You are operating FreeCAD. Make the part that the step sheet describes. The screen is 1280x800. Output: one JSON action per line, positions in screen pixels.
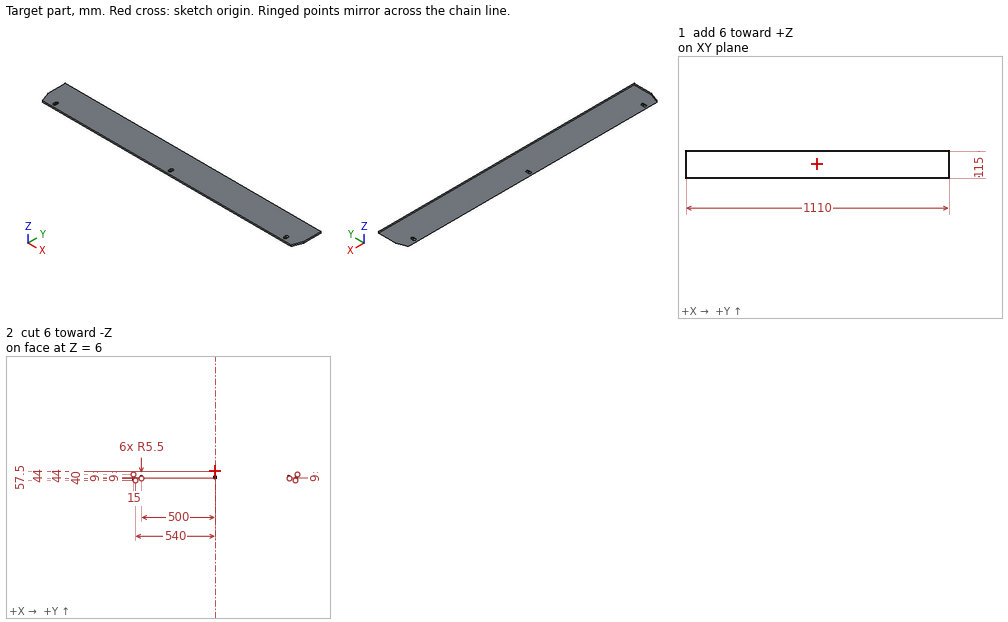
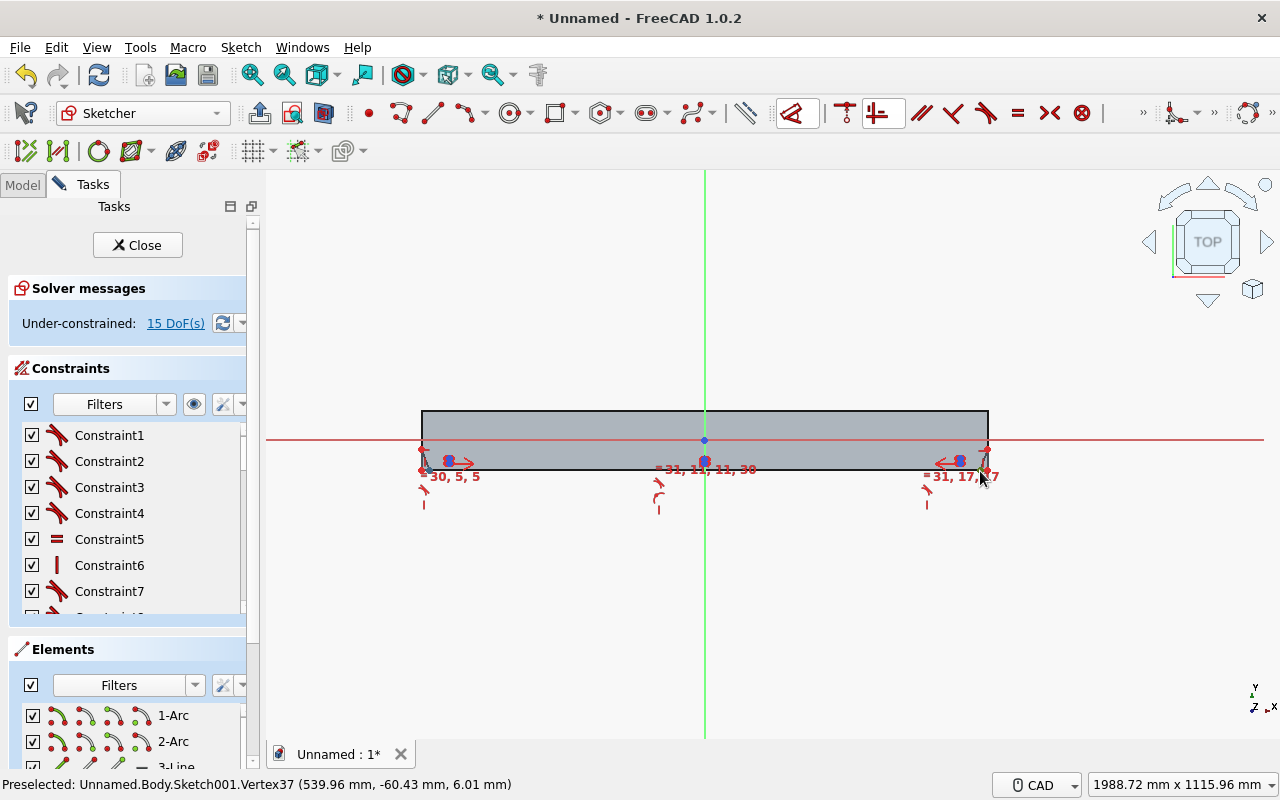
{"action": "left_click", "coordinate": [705, 674]}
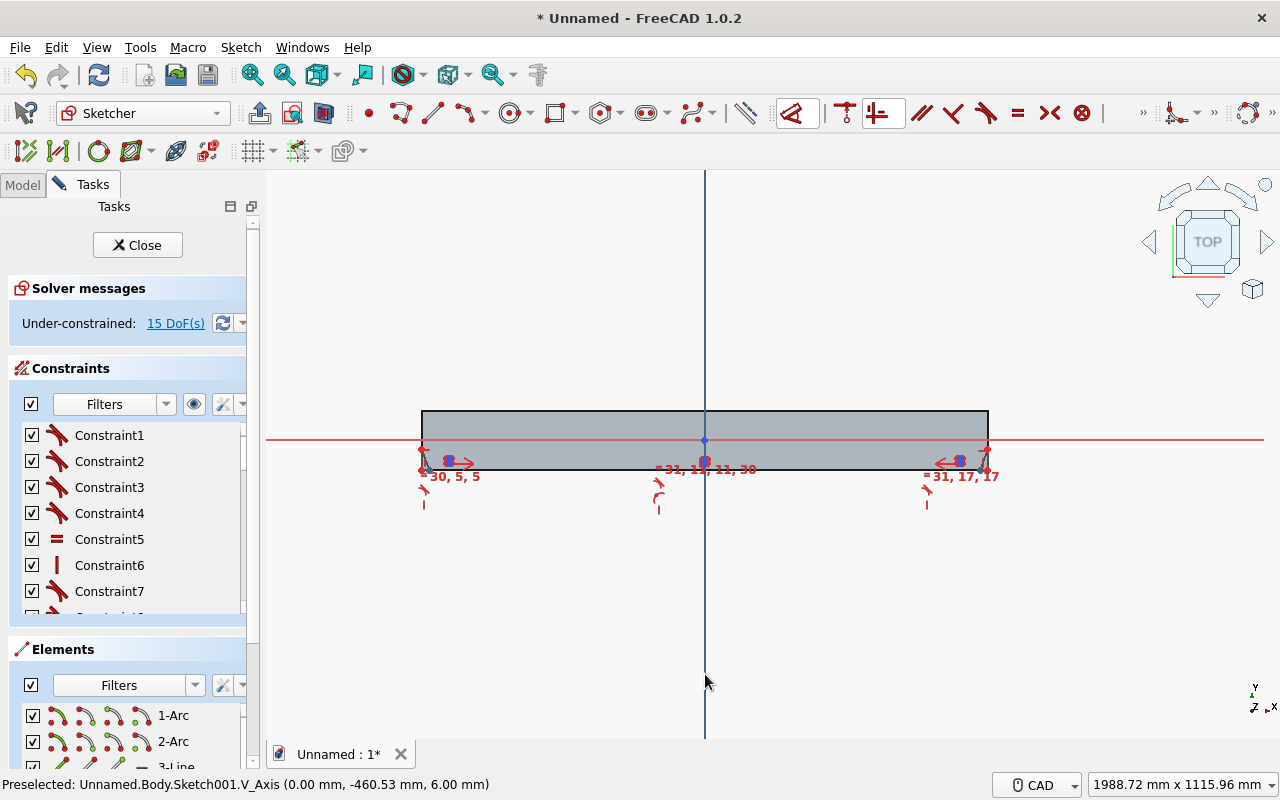
{"action": "key", "text": "s"}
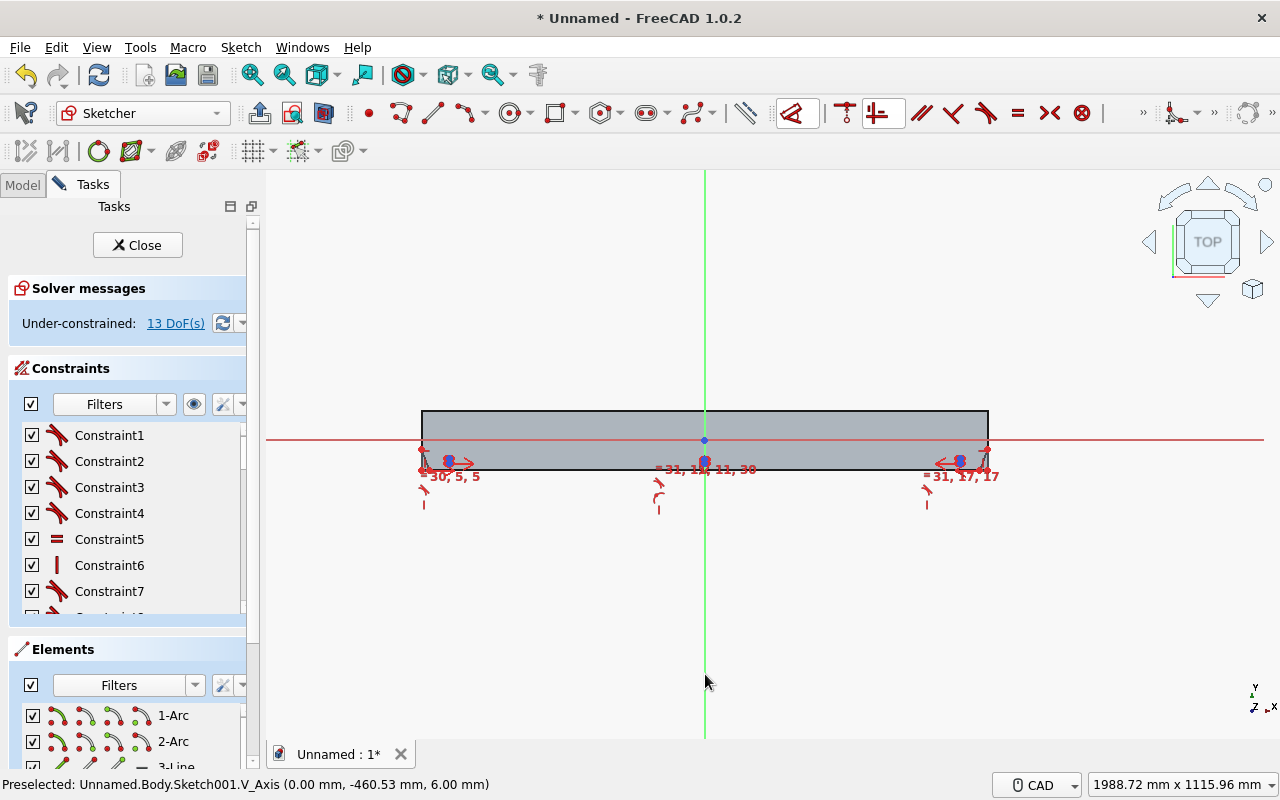
{"action": "left_click", "coordinate": [422, 450]}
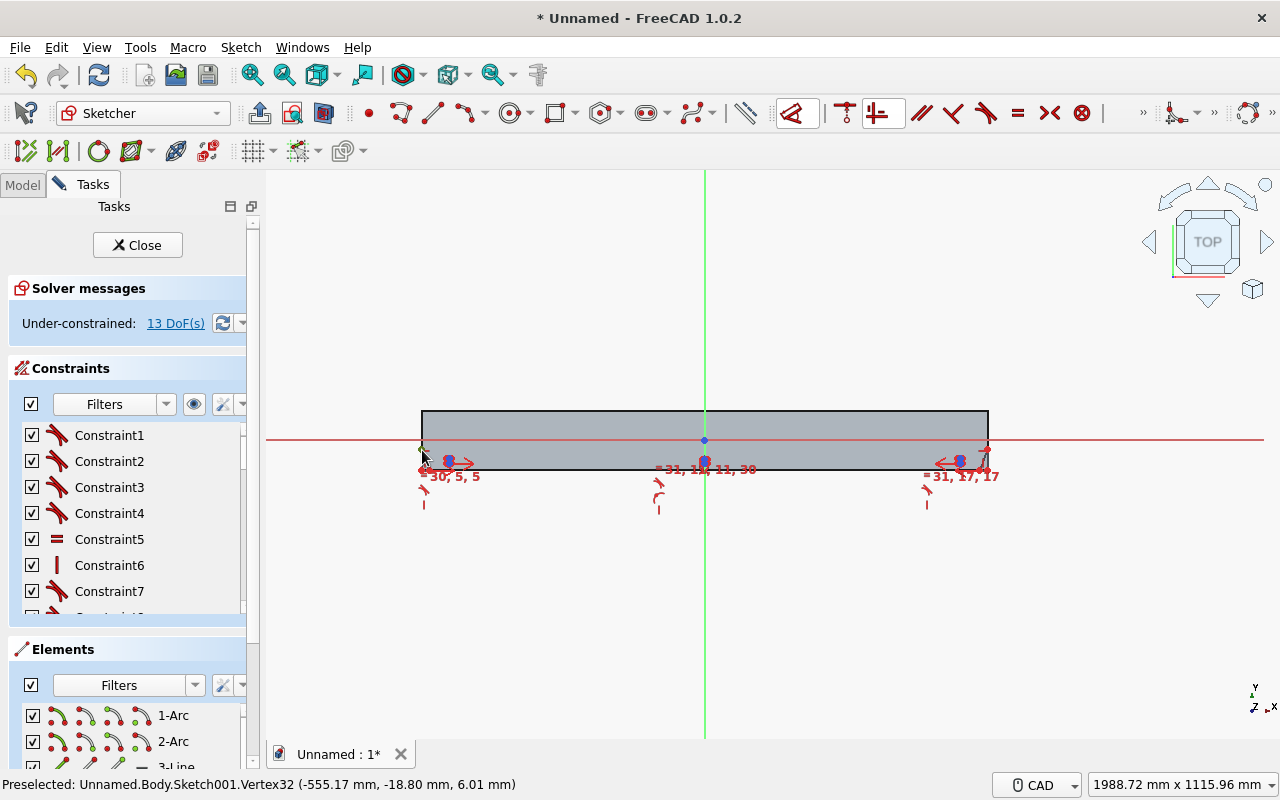
{"action": "left_click", "coordinate": [988, 450]}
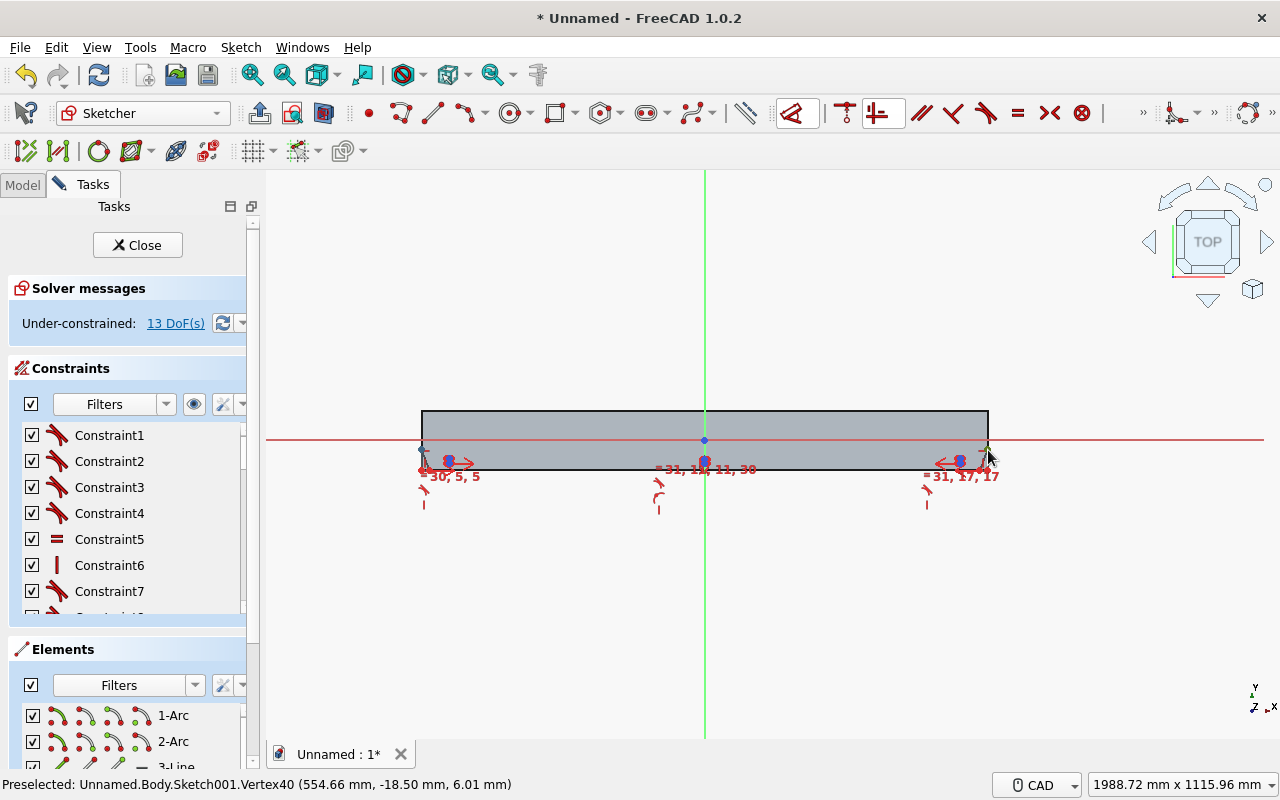
{"action": "left_click", "coordinate": [705, 674]}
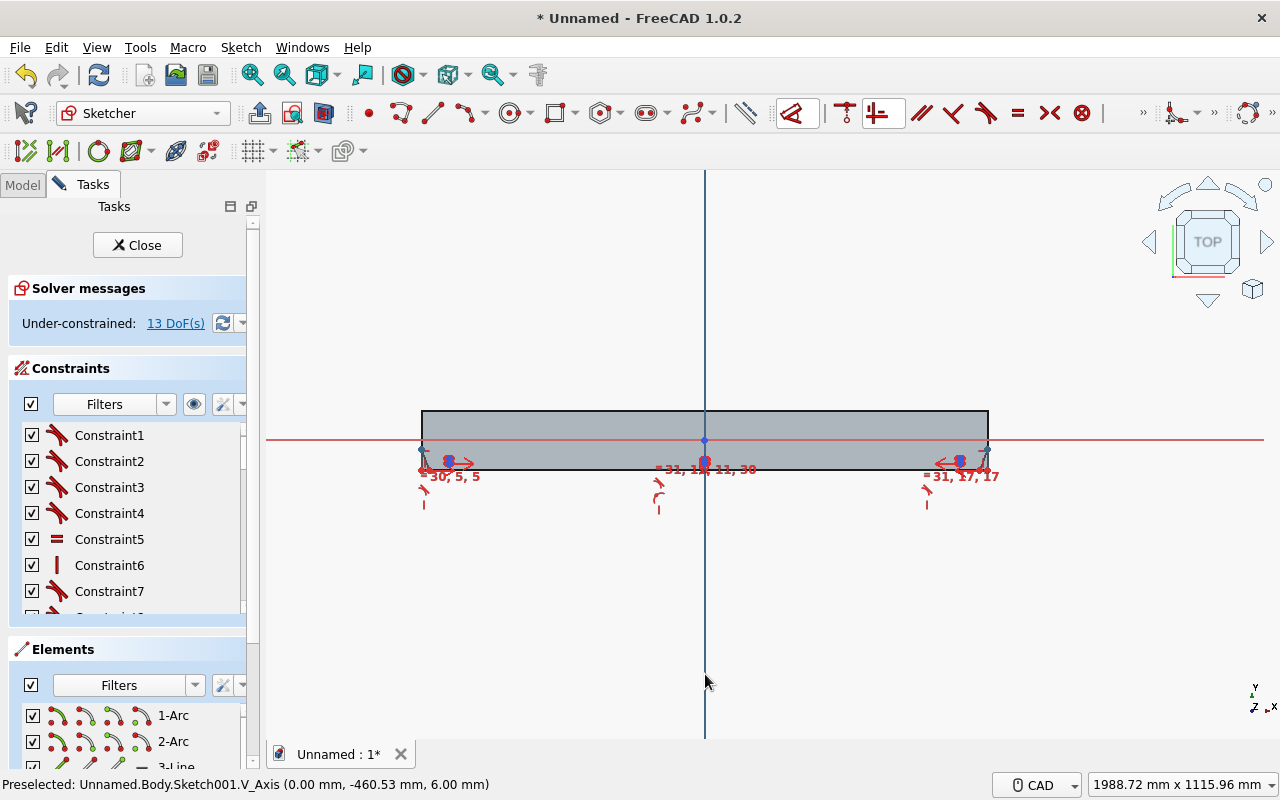
{"action": "left_click", "coordinate": [1050, 114]}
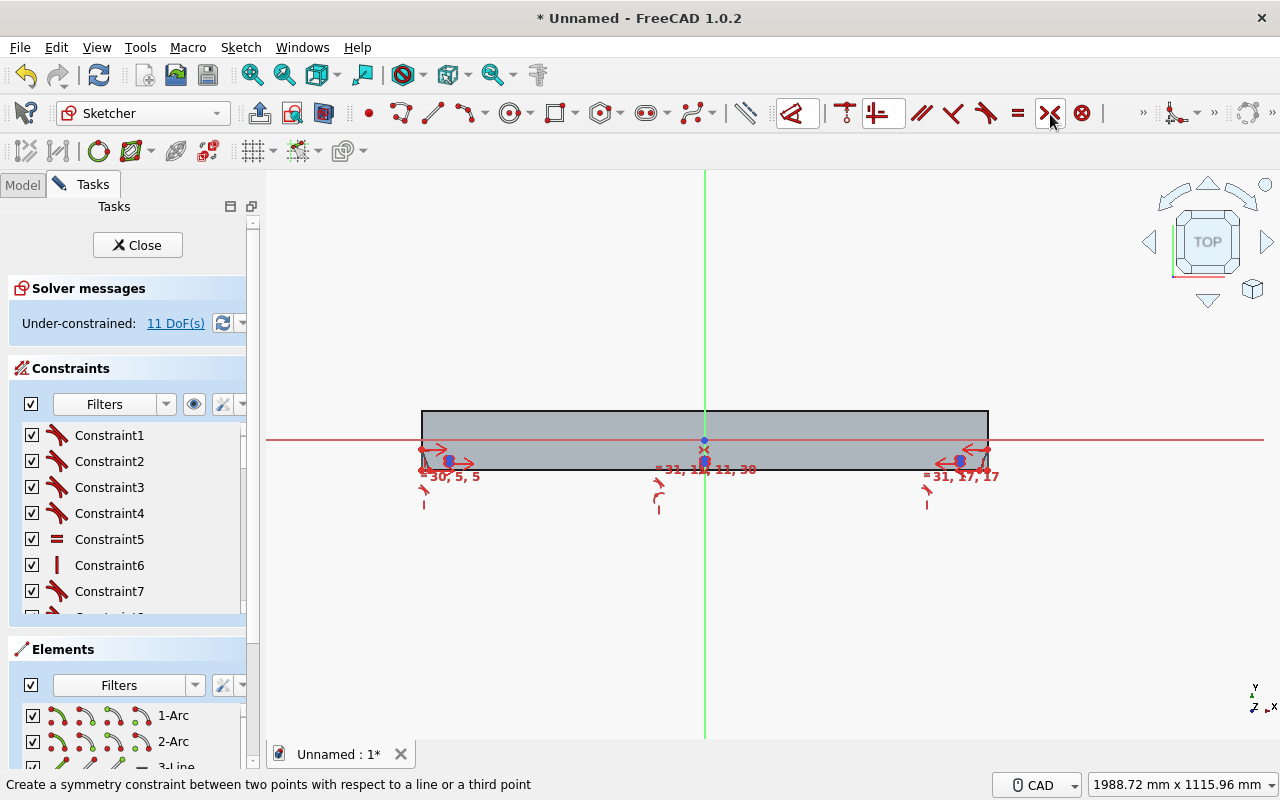
{"action": "left_click", "coordinate": [792, 114]}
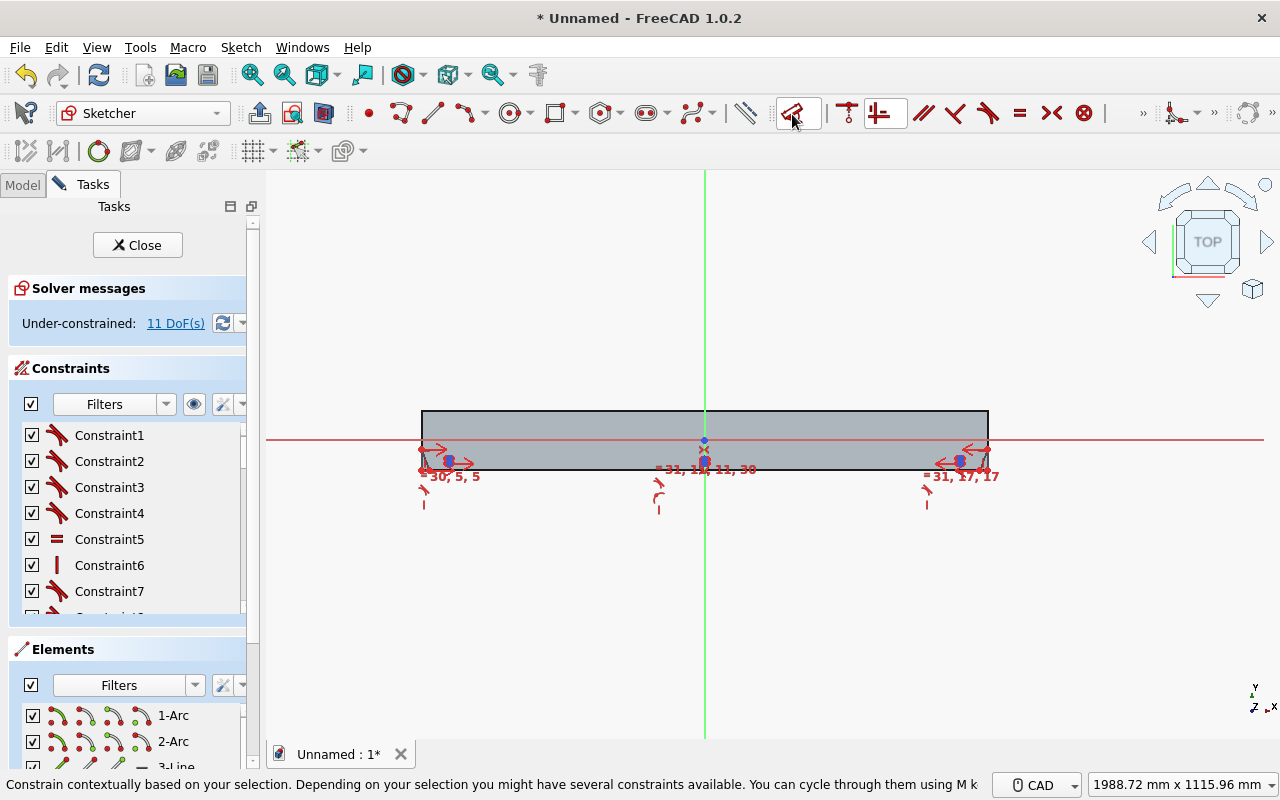
{"action": "scroll", "coordinate": [449, 466], "scroll_direction": "up", "scroll_amount": 14}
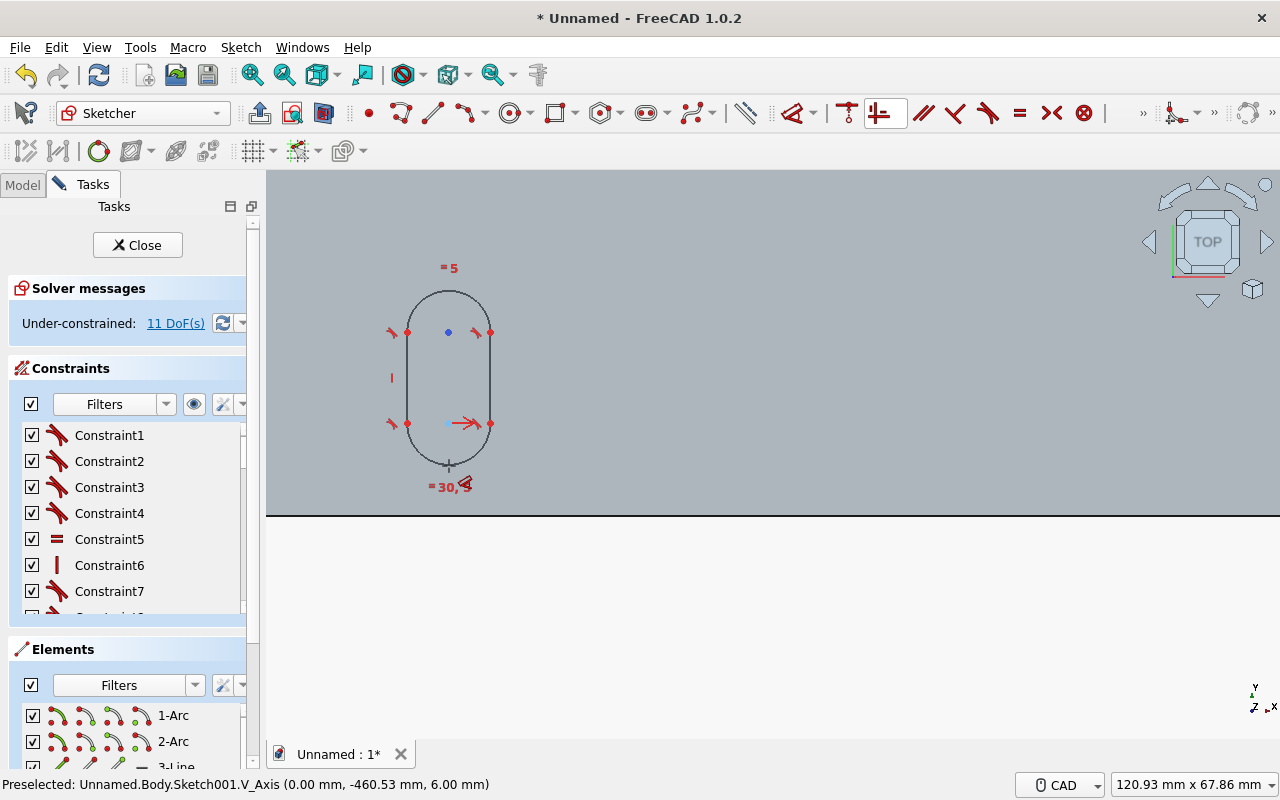
{"action": "left_click", "coordinate": [449, 465]}
{"action": "left_click", "coordinate": [449, 497]}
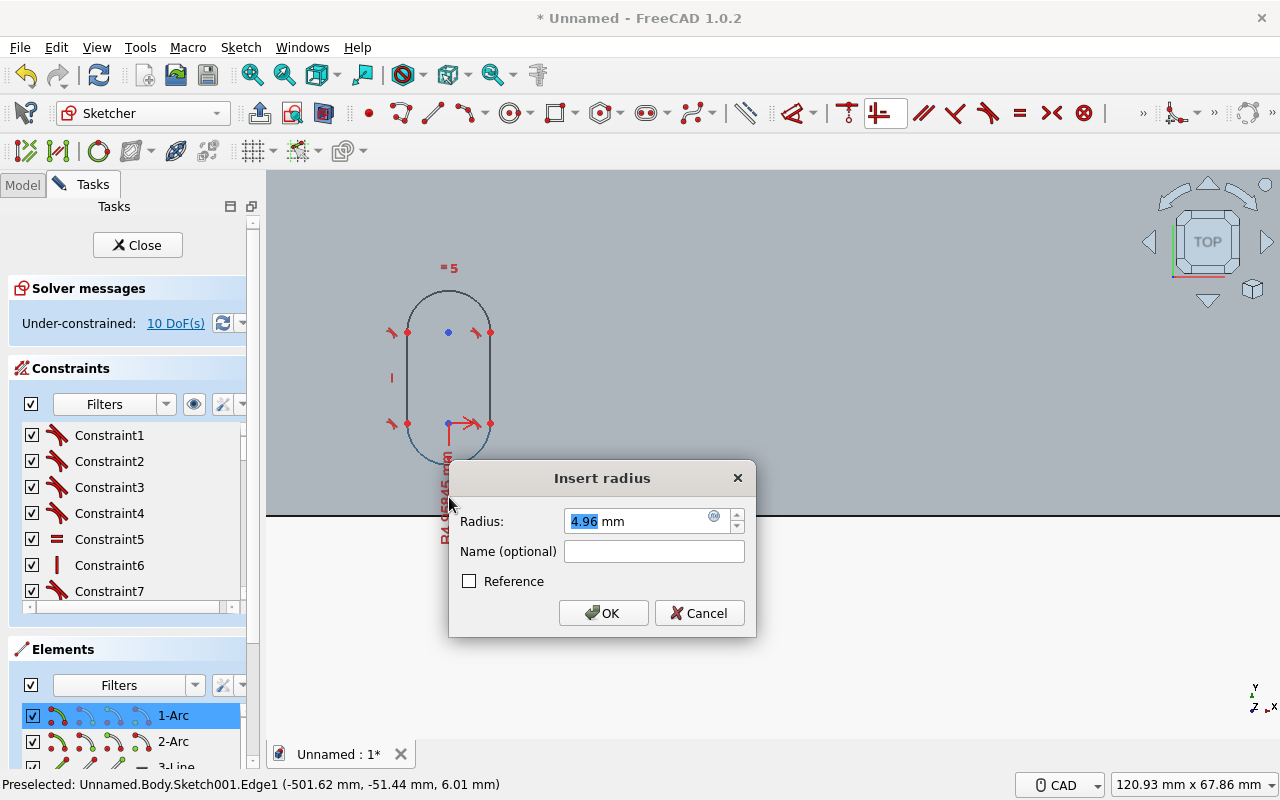
{"action": "type", "text": "5.5"}
{"action": "key", "text": "Return"}